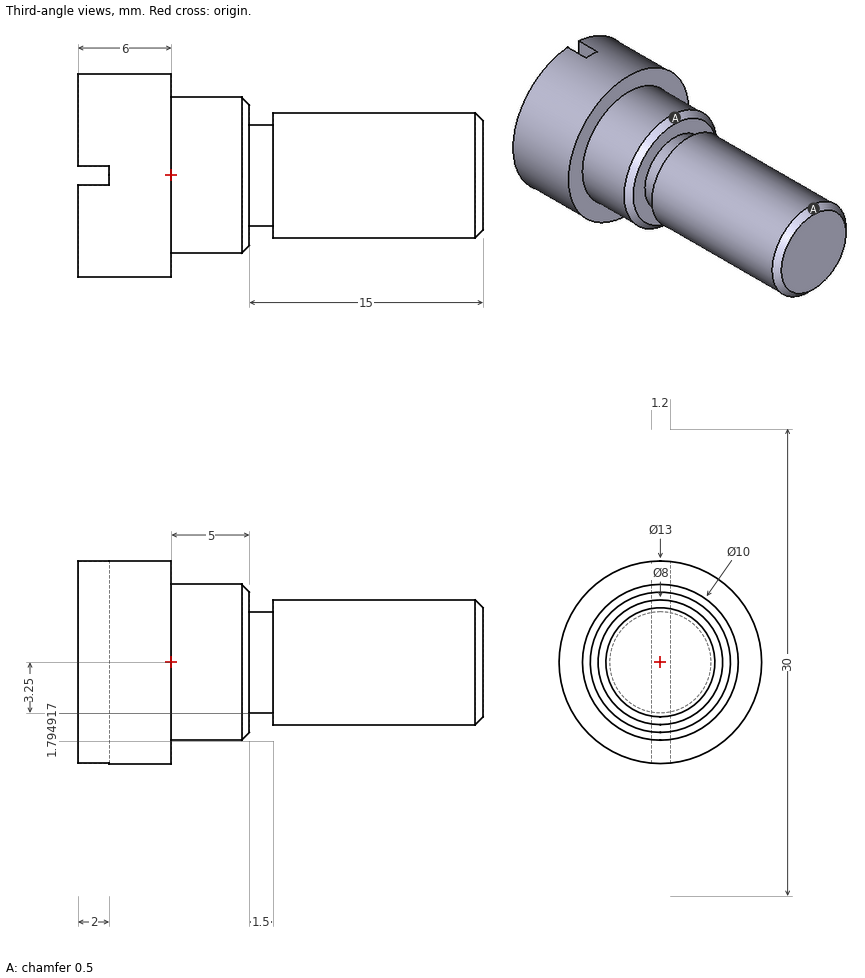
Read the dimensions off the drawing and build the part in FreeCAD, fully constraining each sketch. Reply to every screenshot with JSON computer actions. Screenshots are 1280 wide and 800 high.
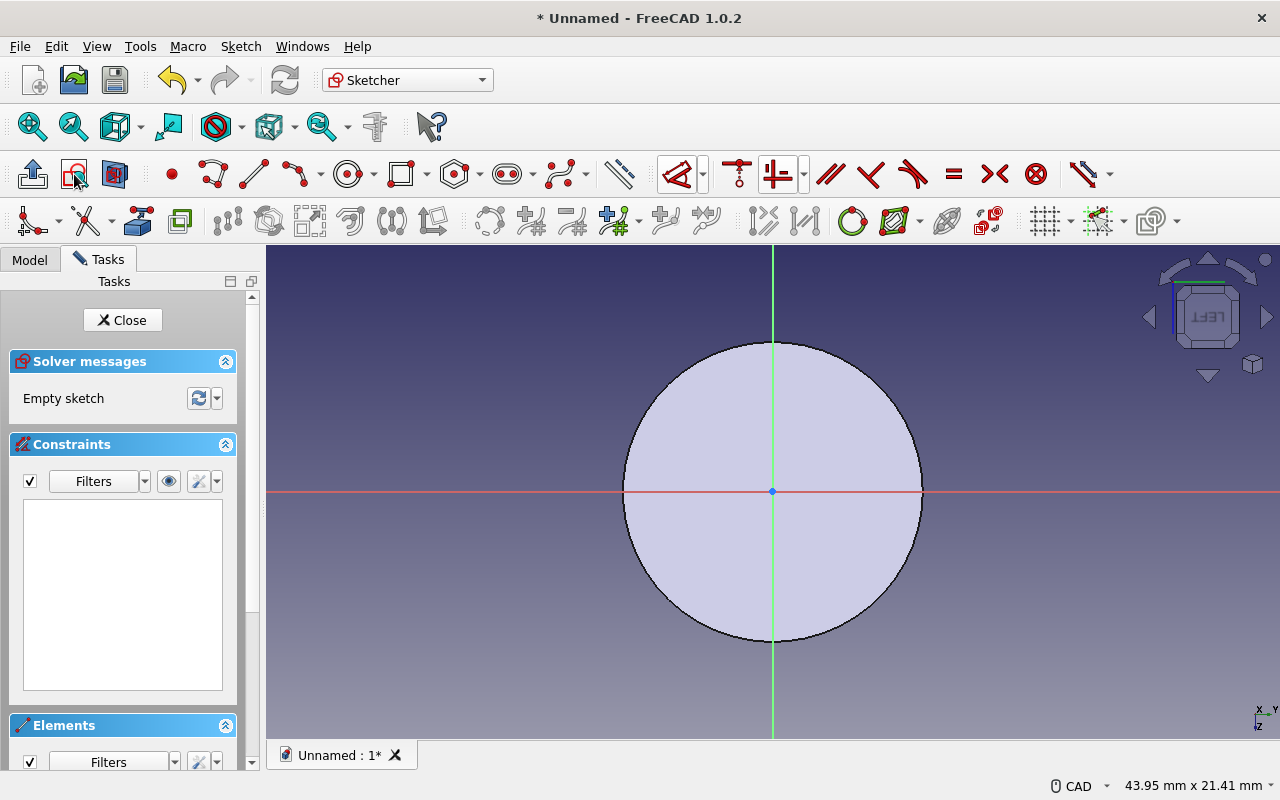
{"action": "scroll", "coordinate": [649, 492], "scroll_direction": "down", "scroll_amount": 4}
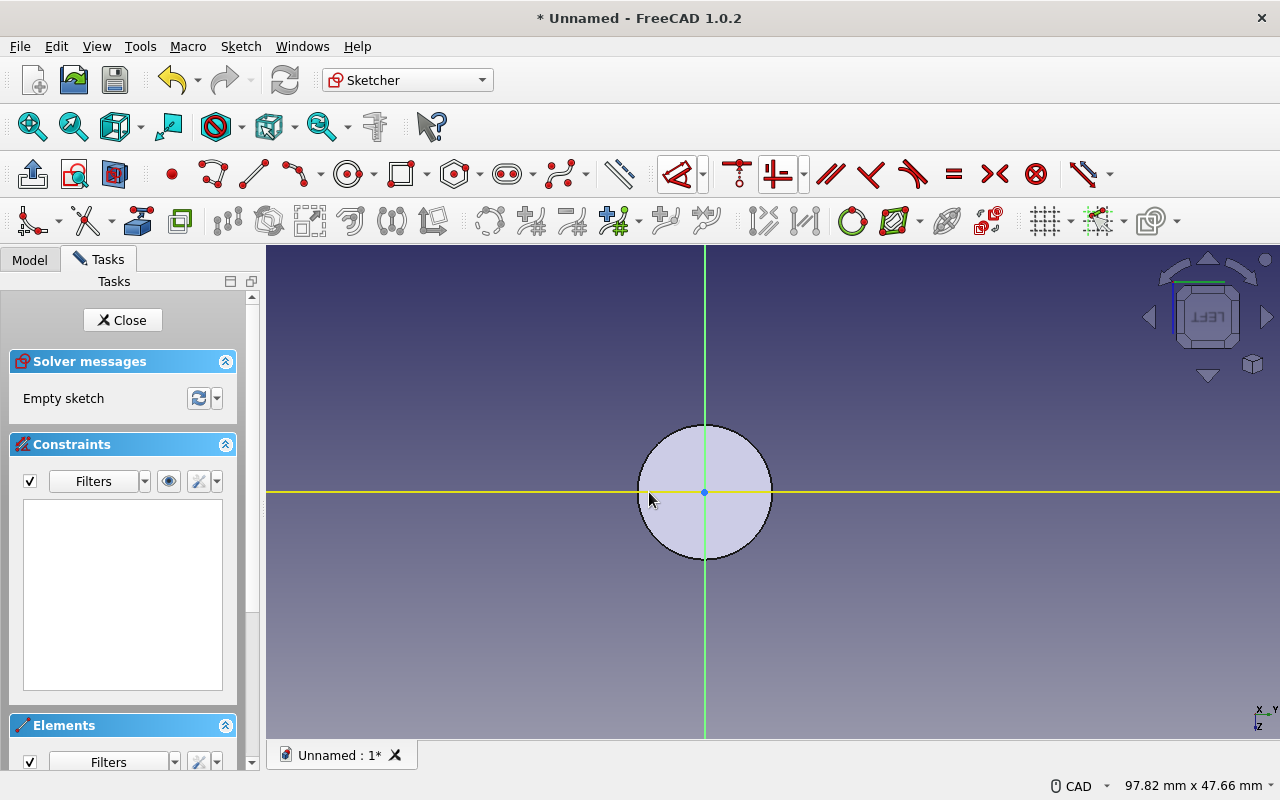
{"action": "left_click", "coordinate": [426, 174]}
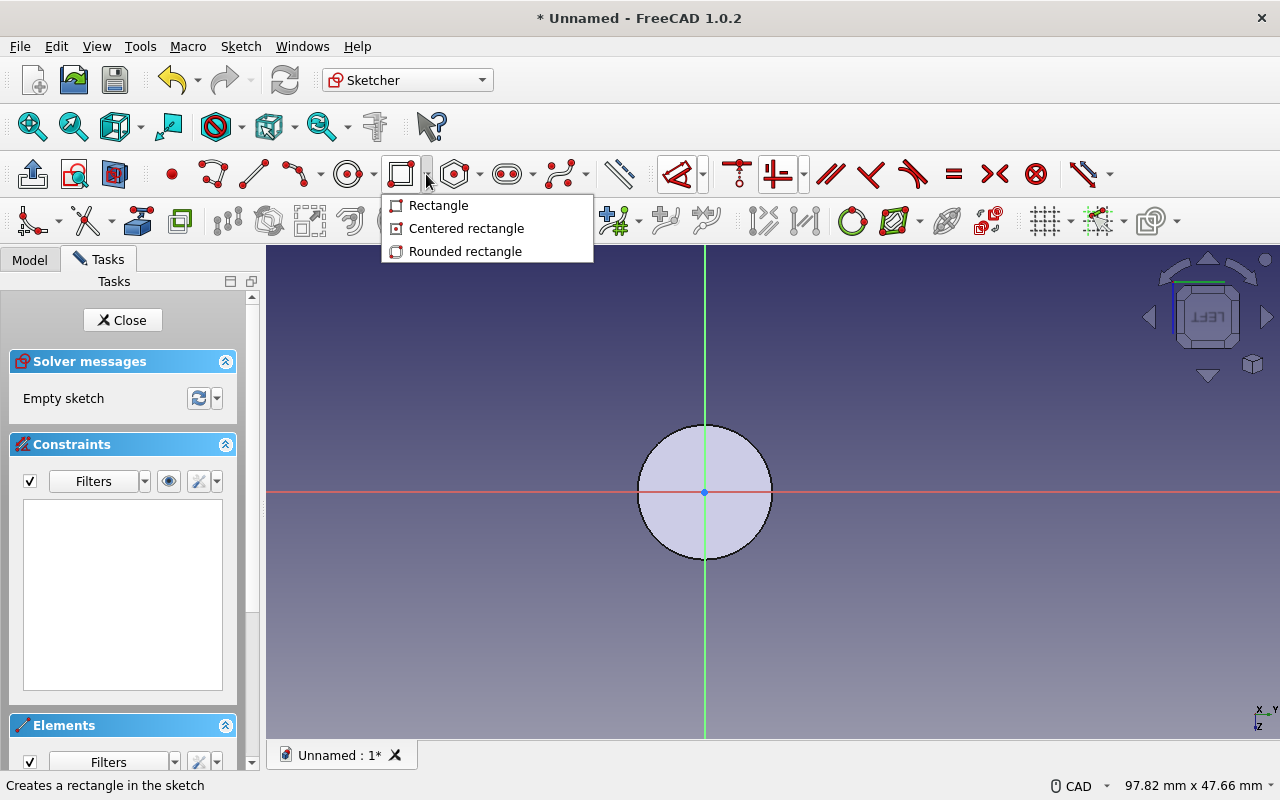
{"action": "left_click", "coordinate": [488, 228]}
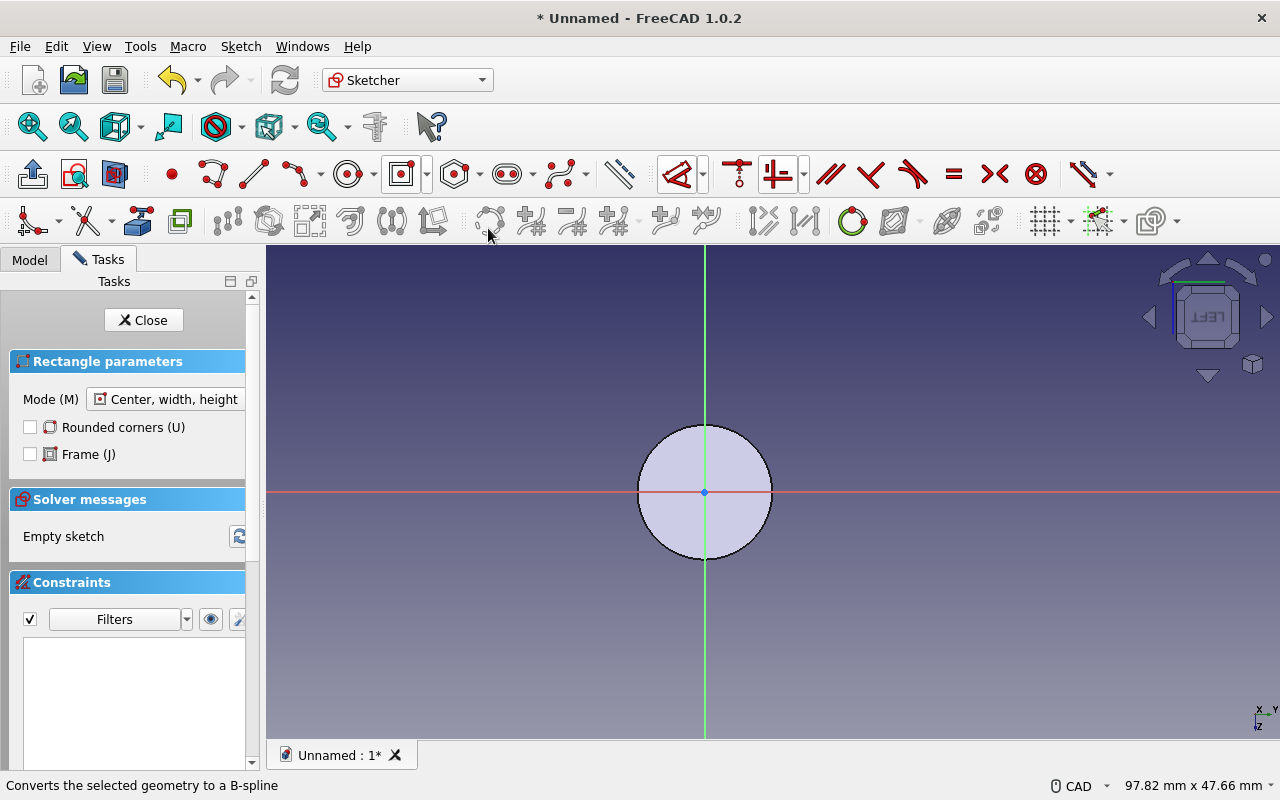
{"action": "scroll", "coordinate": [705, 492], "scroll_direction": "up", "scroll_amount": 5}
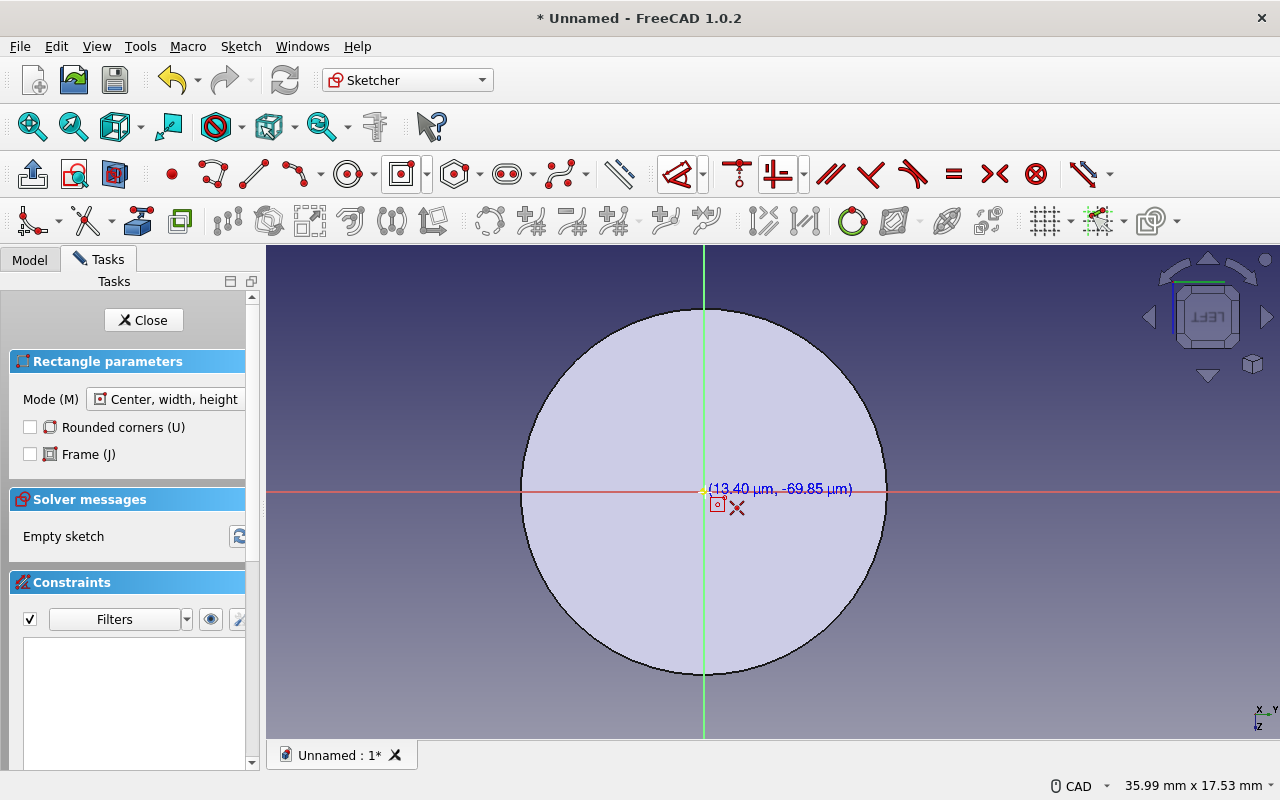
{"action": "left_click", "coordinate": [704, 492]}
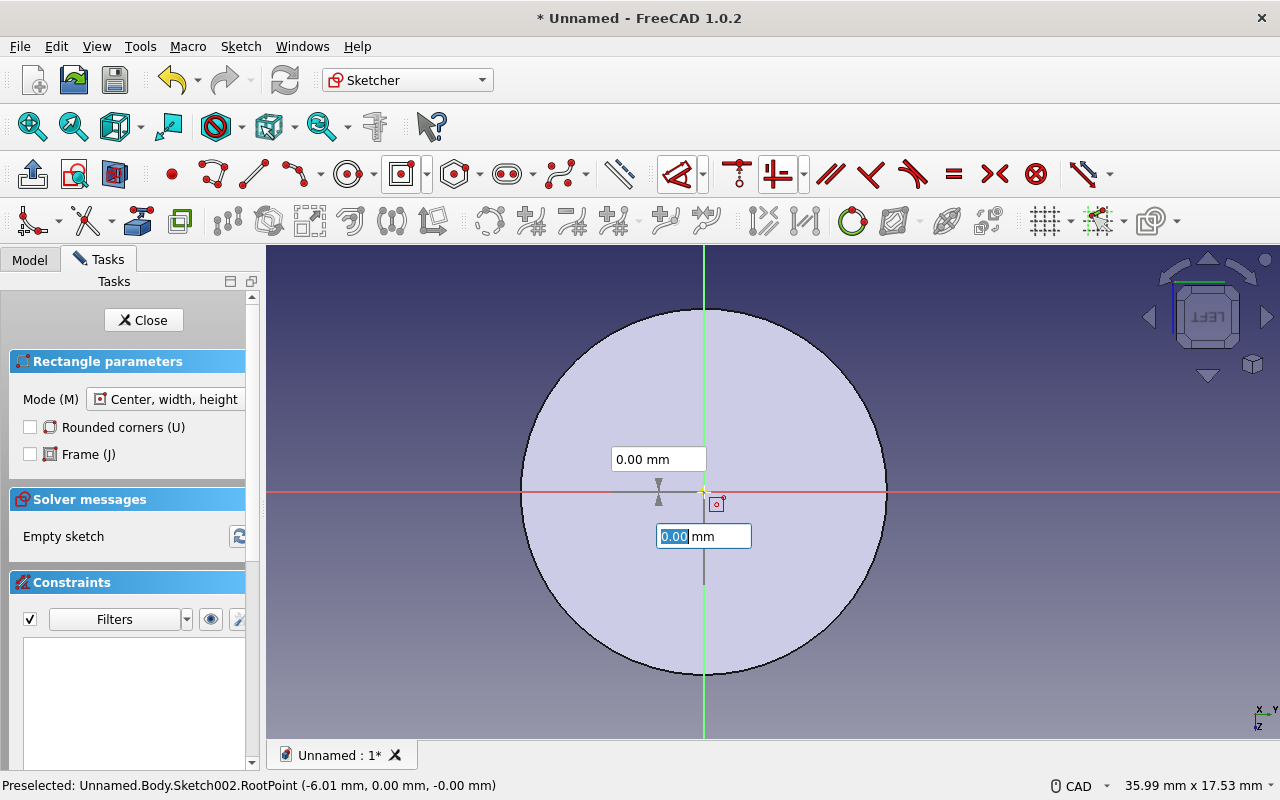
{"action": "scroll", "coordinate": [705, 492], "scroll_direction": "down", "scroll_amount": 5}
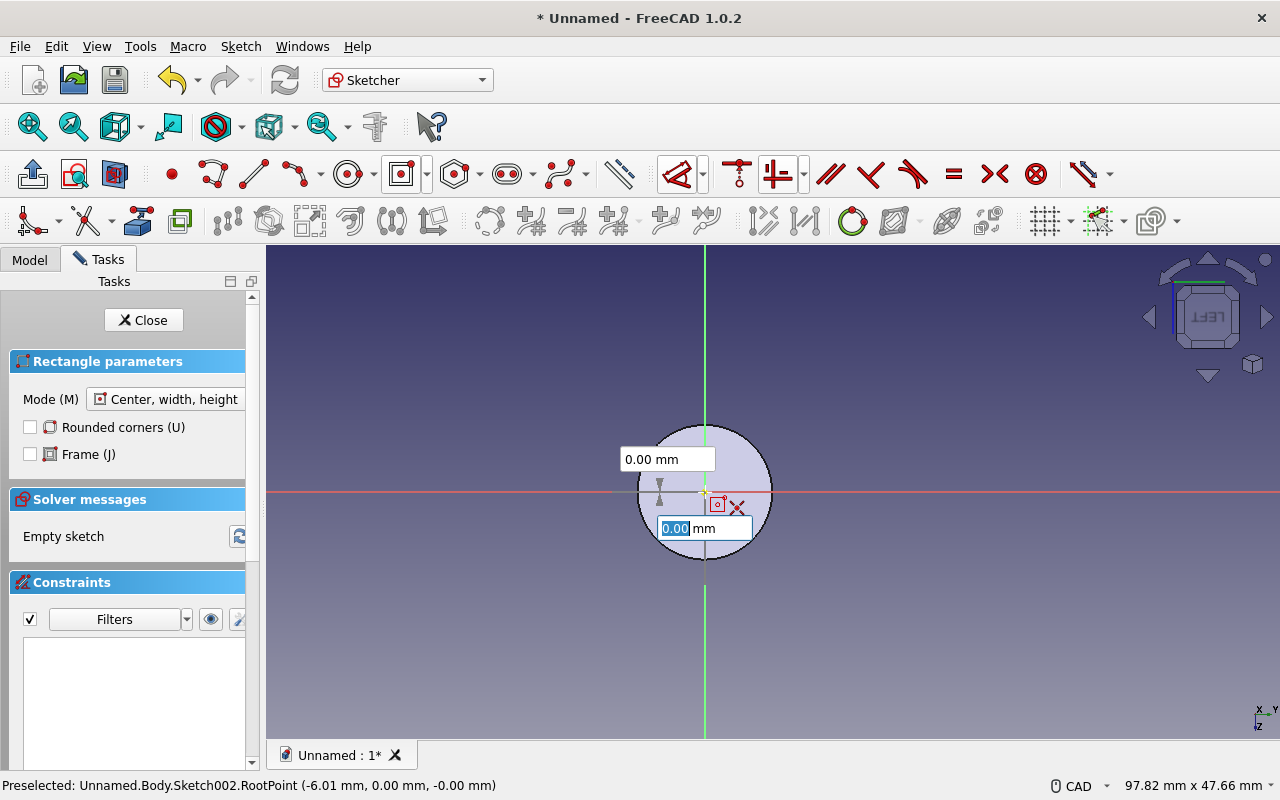
{"action": "scroll", "coordinate": [711, 337], "scroll_direction": "up", "scroll_amount": 5}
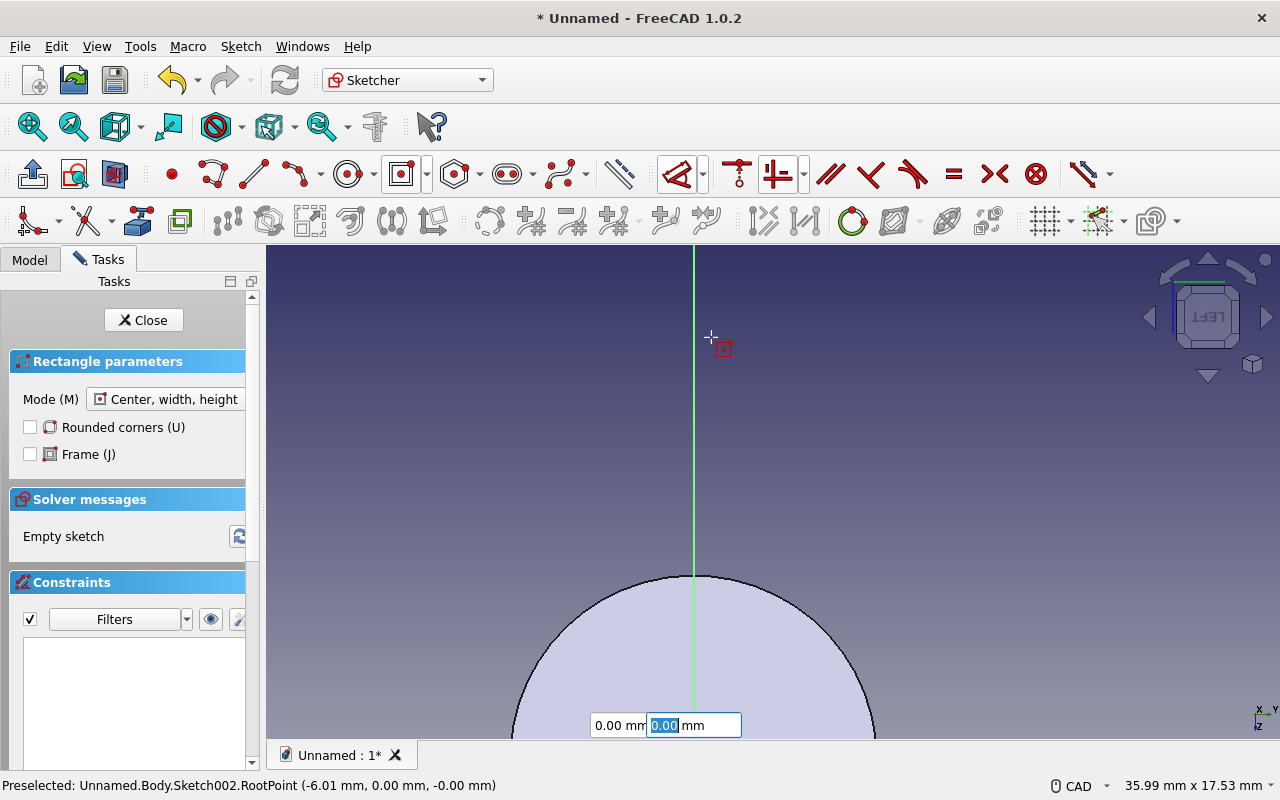
{"action": "left_click", "coordinate": [710, 336]}
{"action": "key", "text": "Escape"}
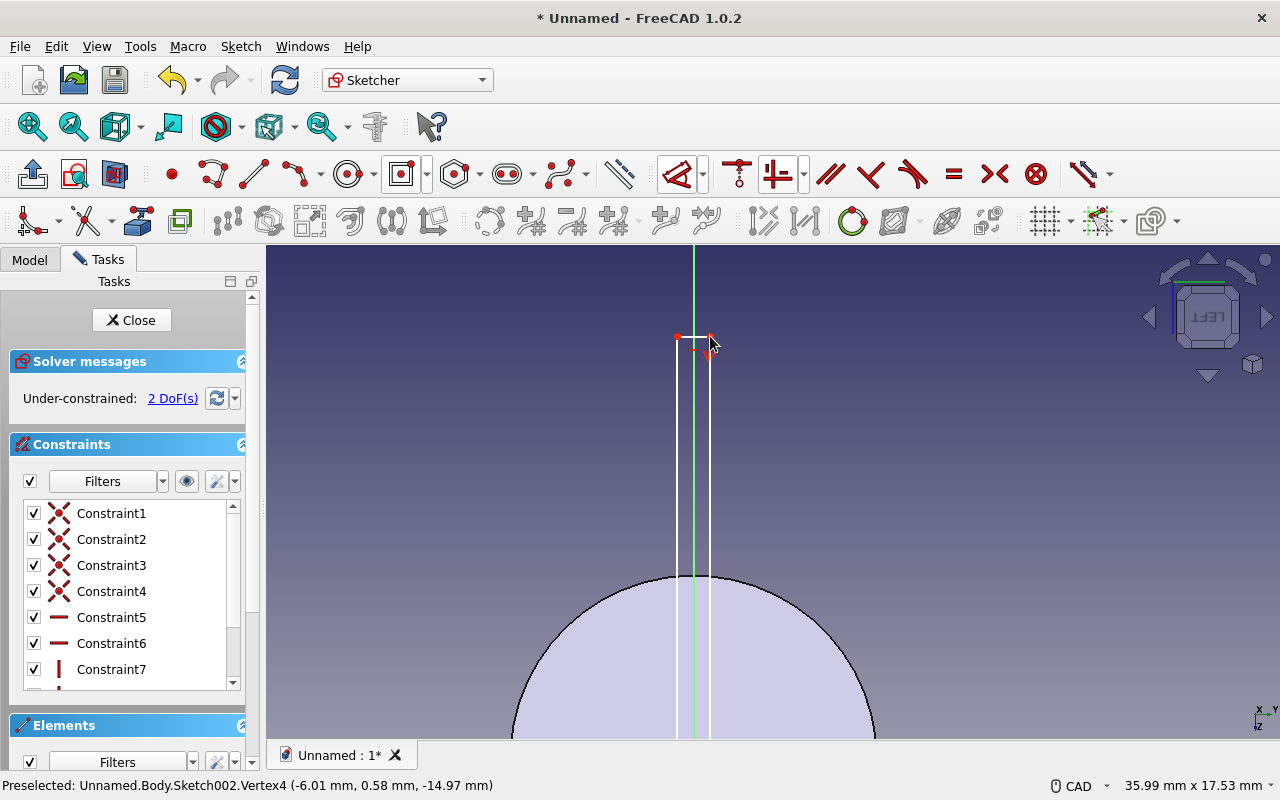
{"action": "key", "text": "d"}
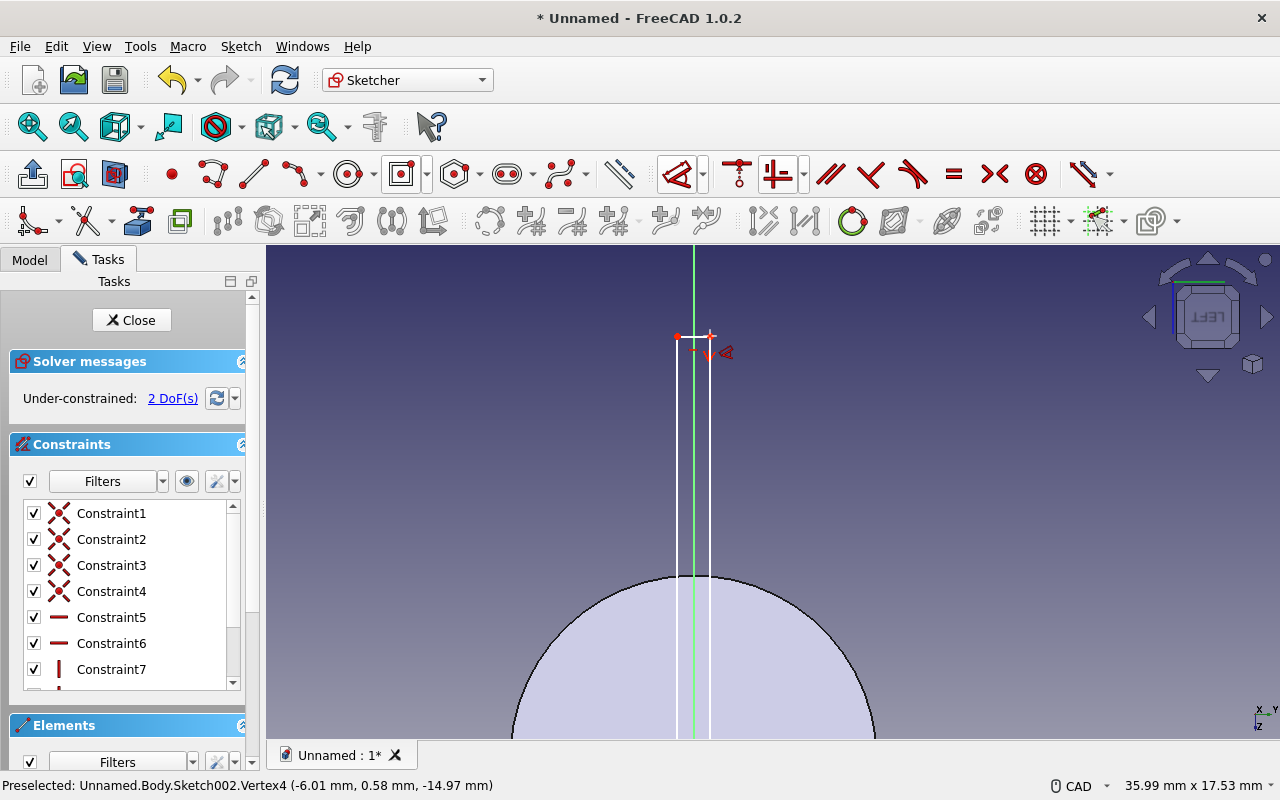
{"action": "left_click", "coordinate": [710, 590]}
{"action": "left_click", "coordinate": [744, 524]}